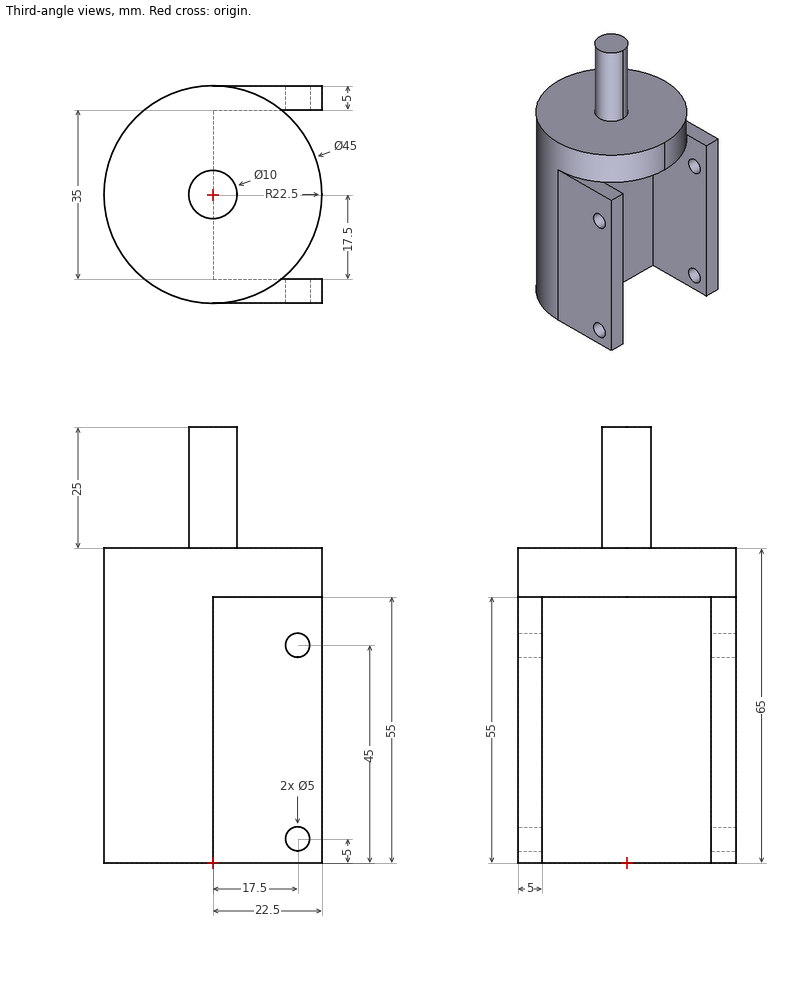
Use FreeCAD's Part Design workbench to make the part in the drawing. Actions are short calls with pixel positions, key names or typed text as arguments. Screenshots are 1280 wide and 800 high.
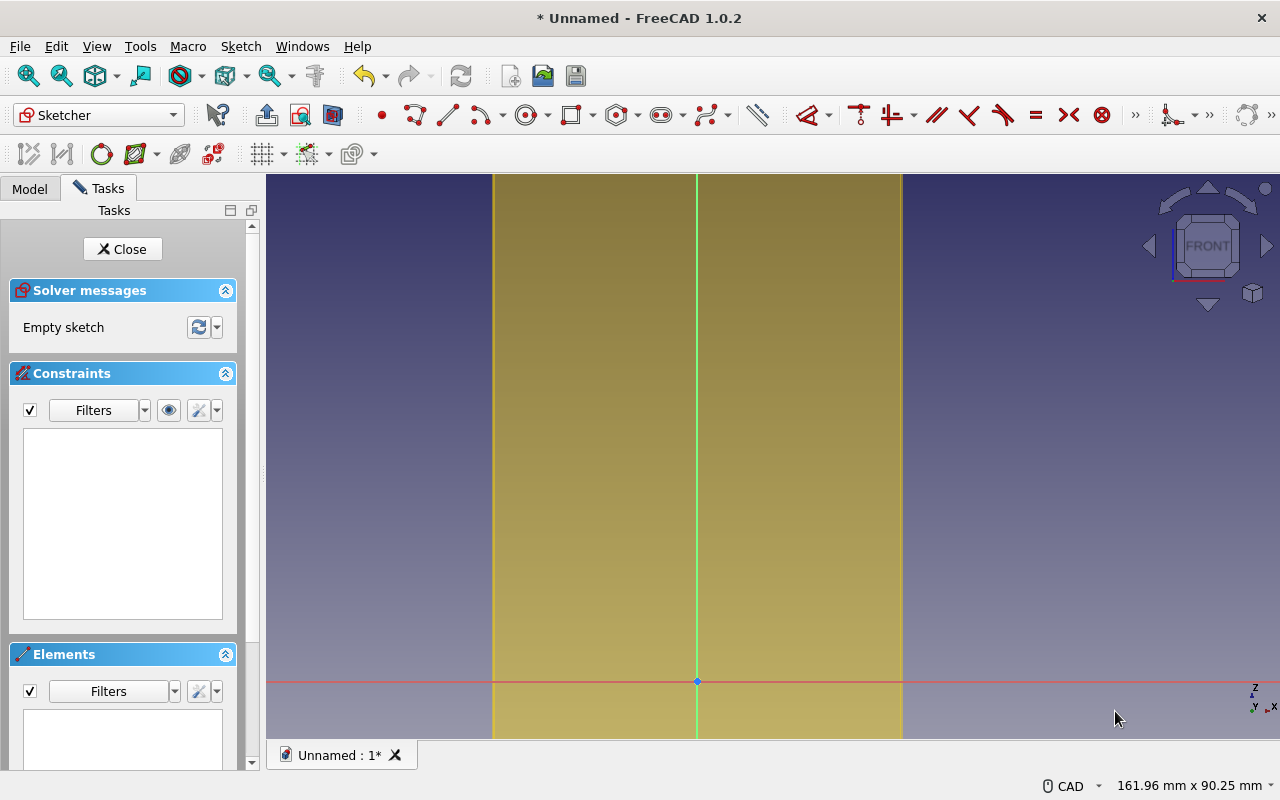
click(570, 116)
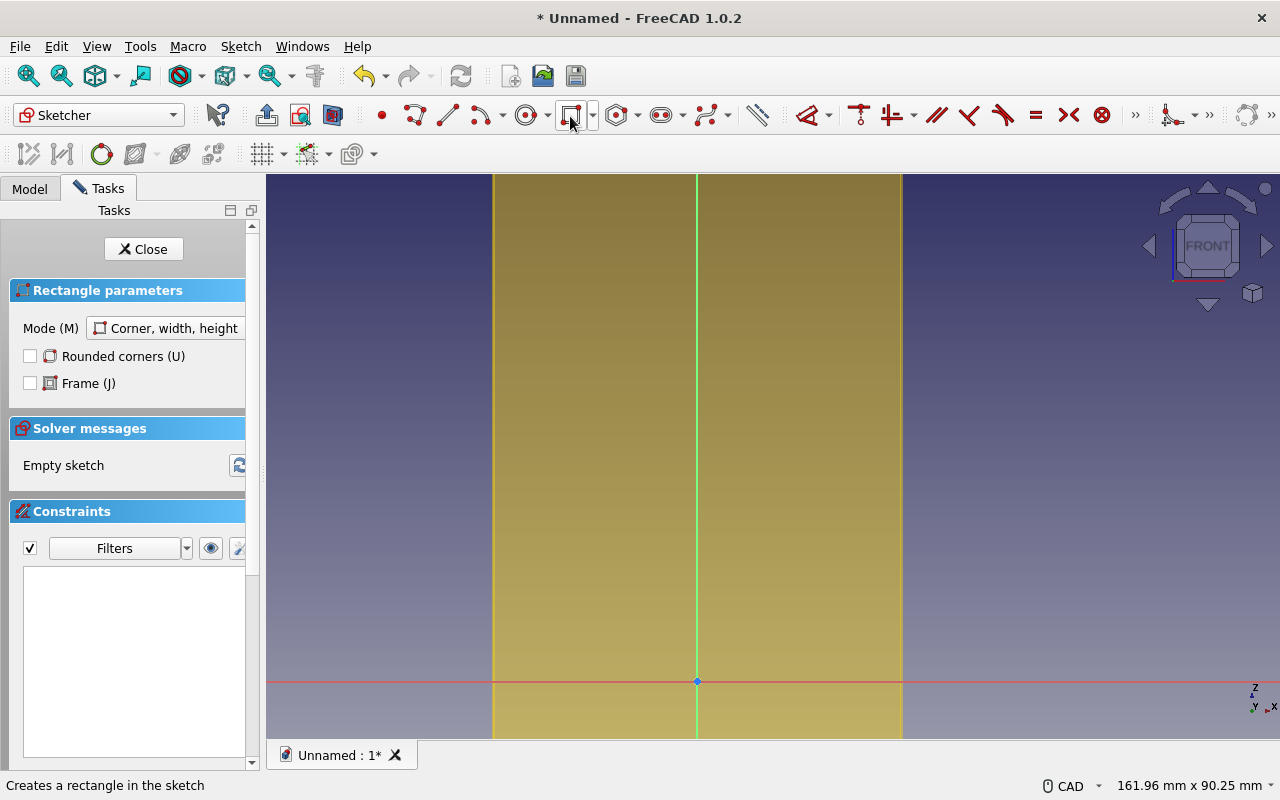
click(697, 682)
click(838, 337)
key(Escape)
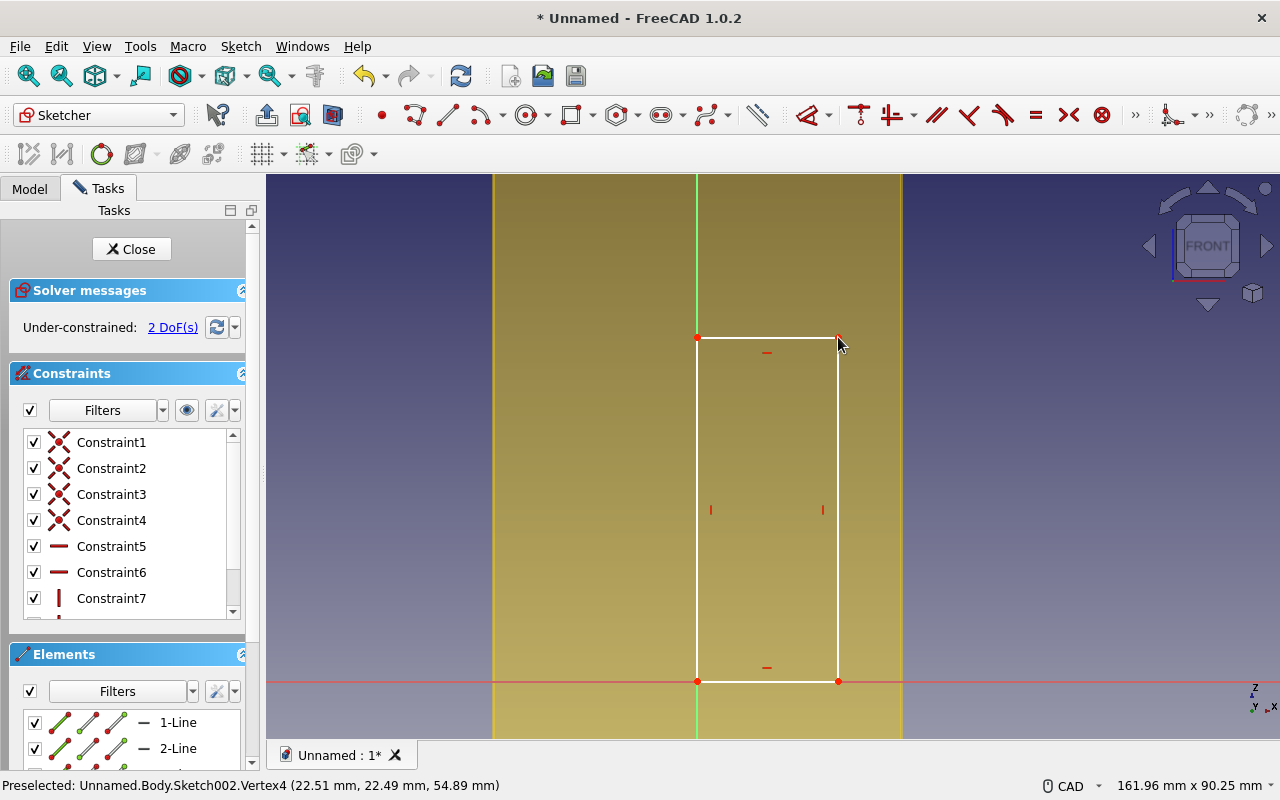
click(806, 116)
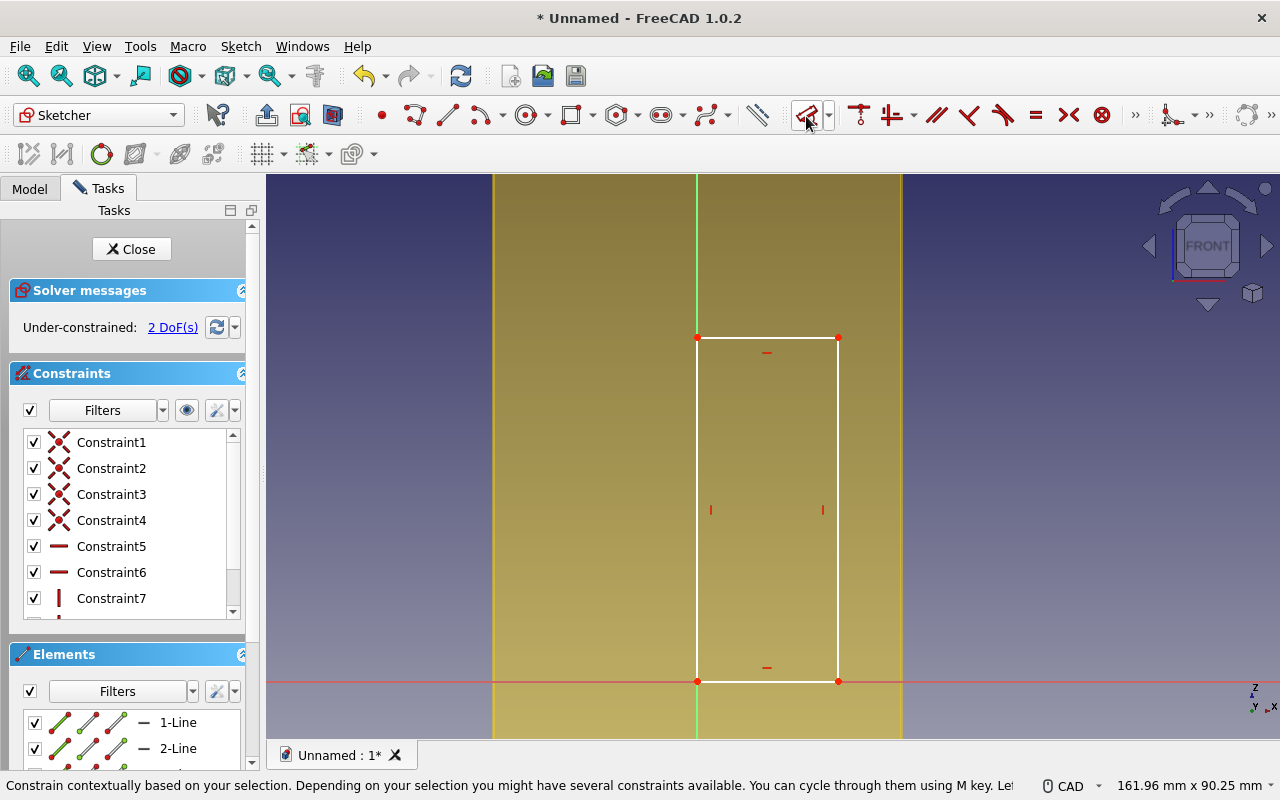
click(838, 579)
click(872, 510)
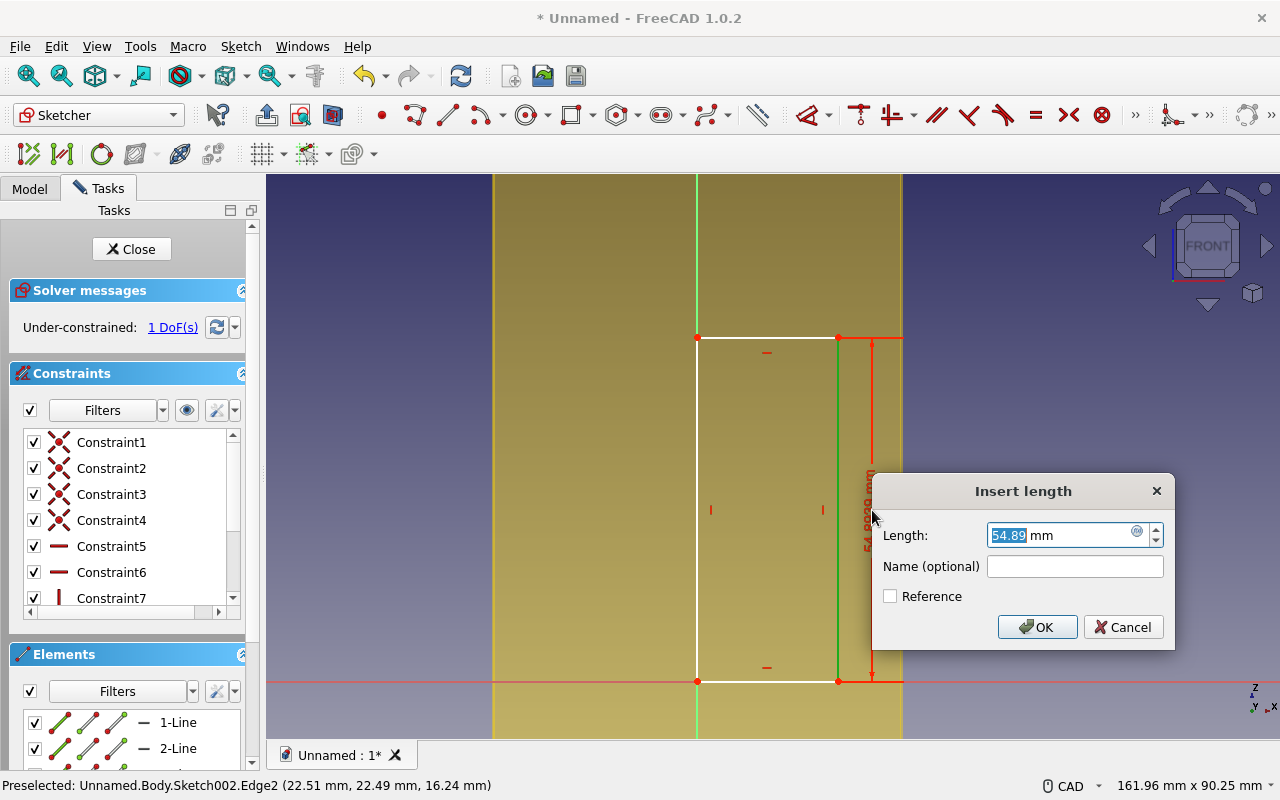
text(55)
key(Return)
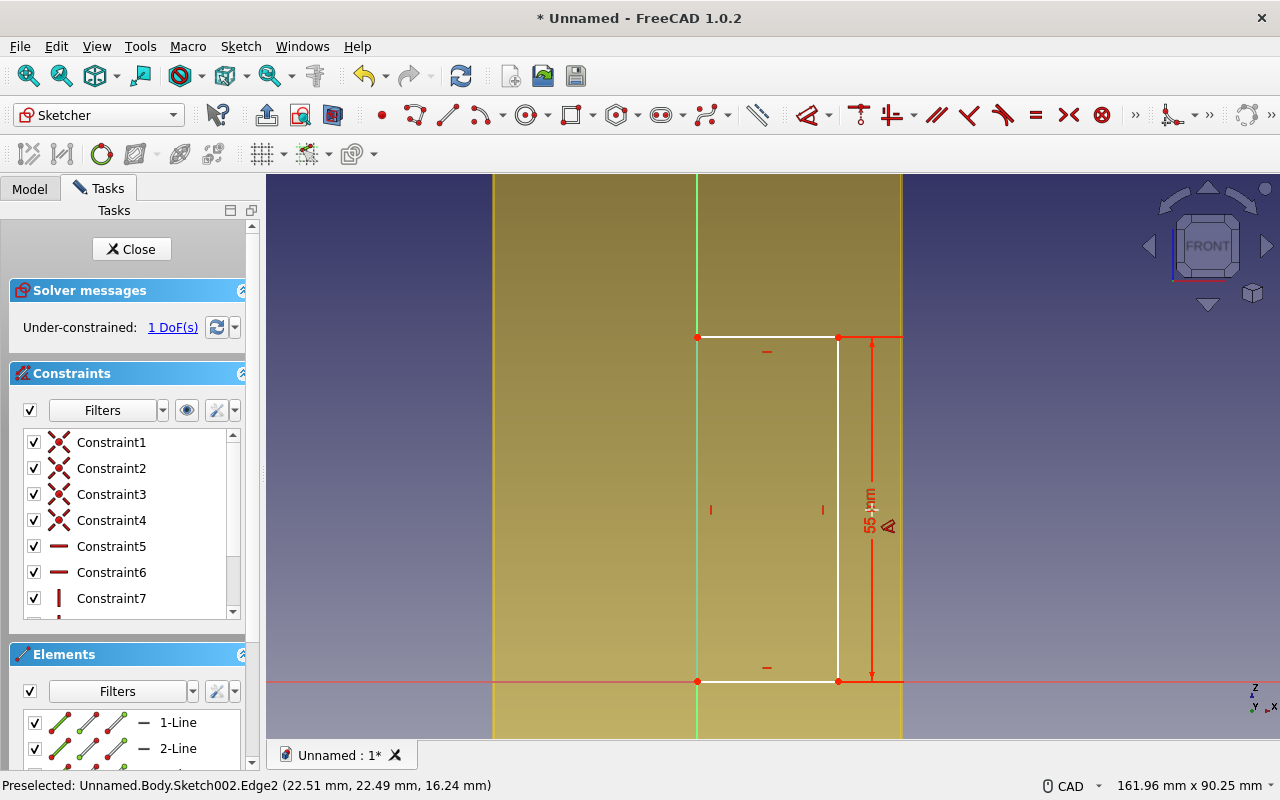
click(739, 682)
click(768, 648)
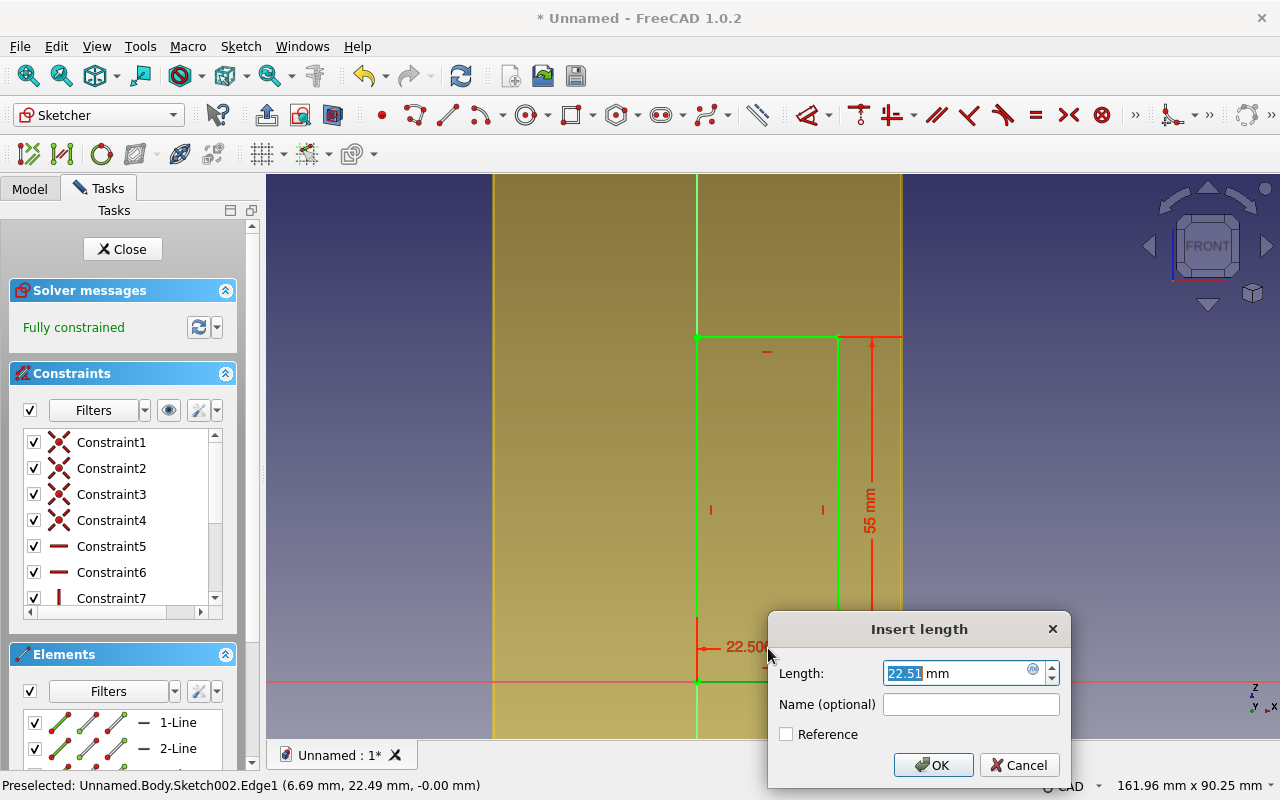
text(22.5)
key(Return)
key(Escape)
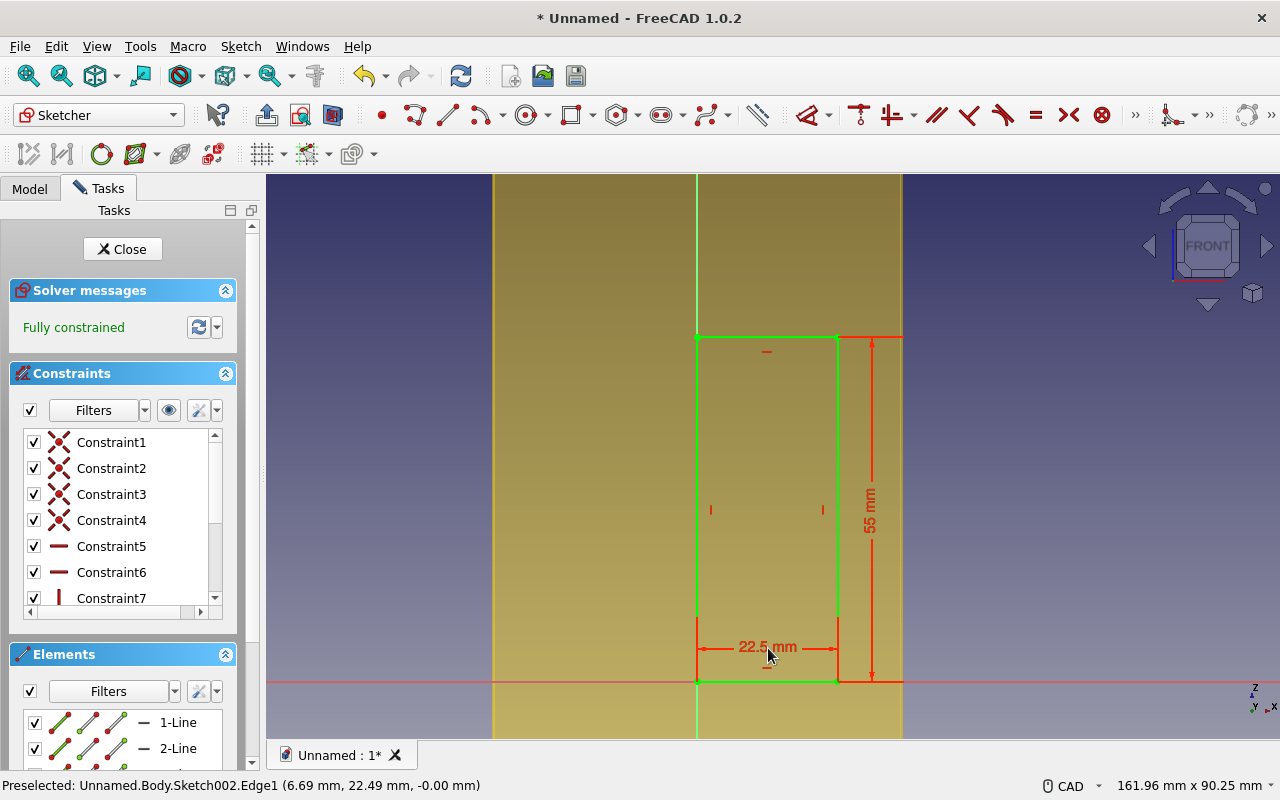
click(123, 249)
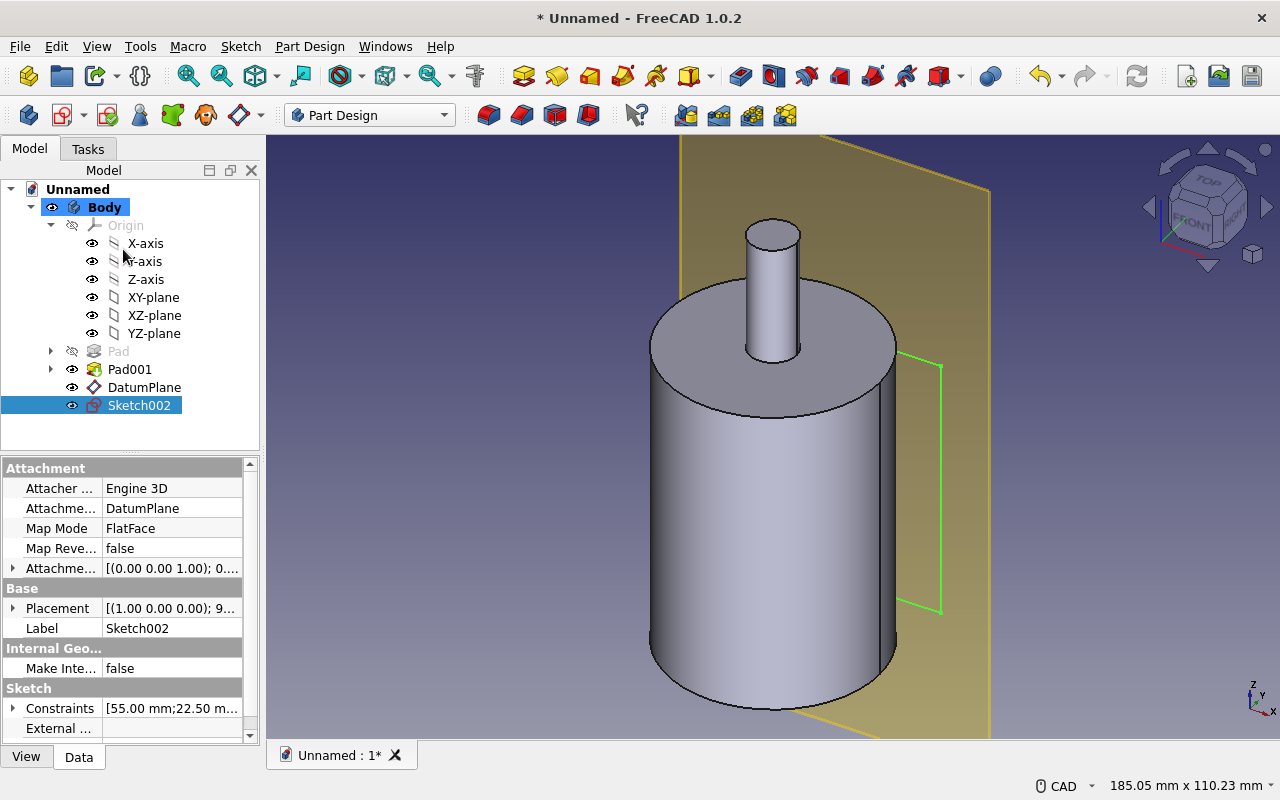
click(524, 76)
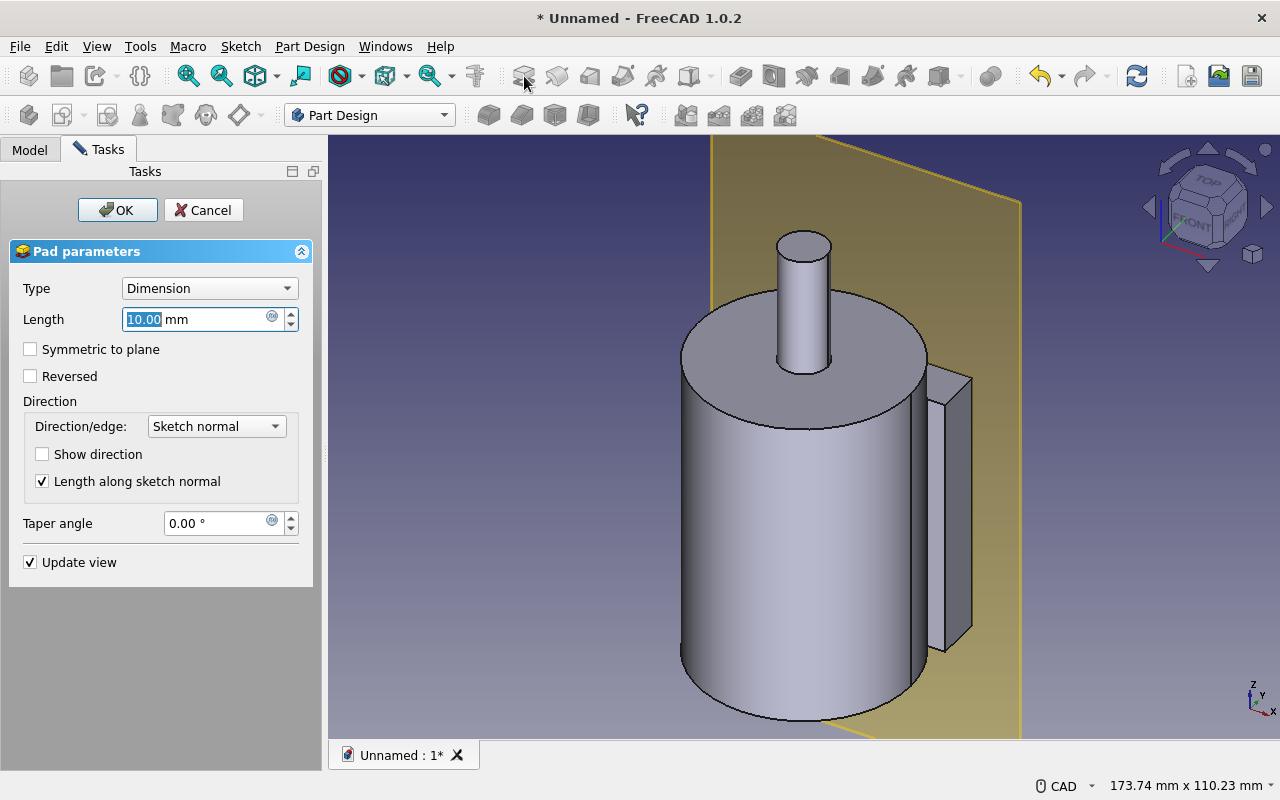
text(5)
key(Tab)